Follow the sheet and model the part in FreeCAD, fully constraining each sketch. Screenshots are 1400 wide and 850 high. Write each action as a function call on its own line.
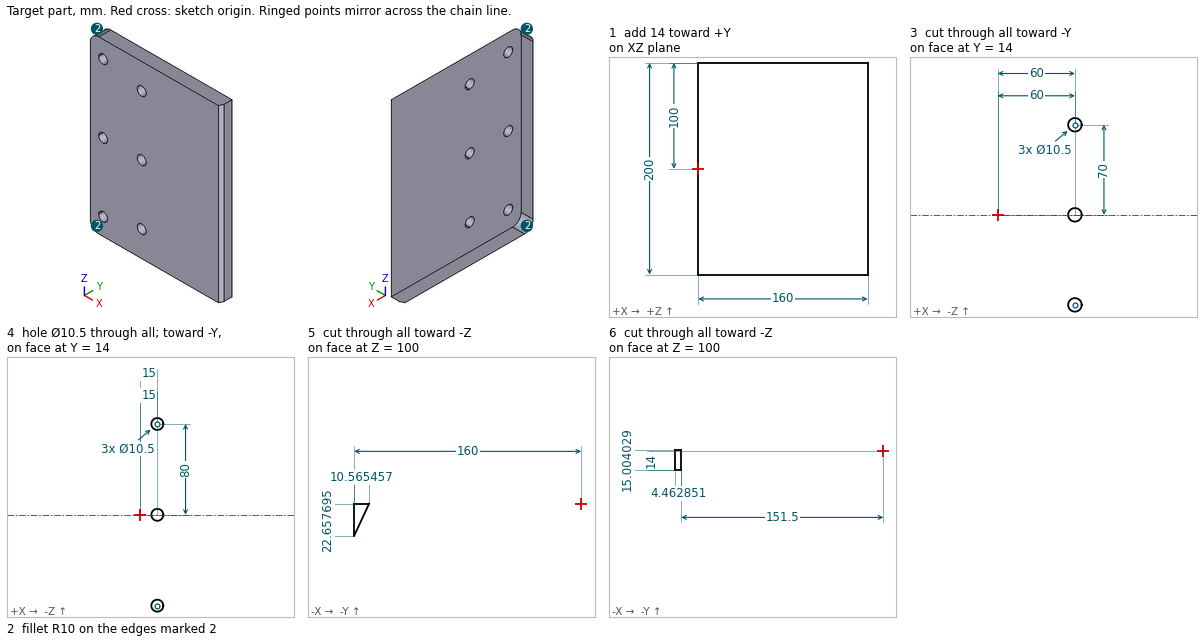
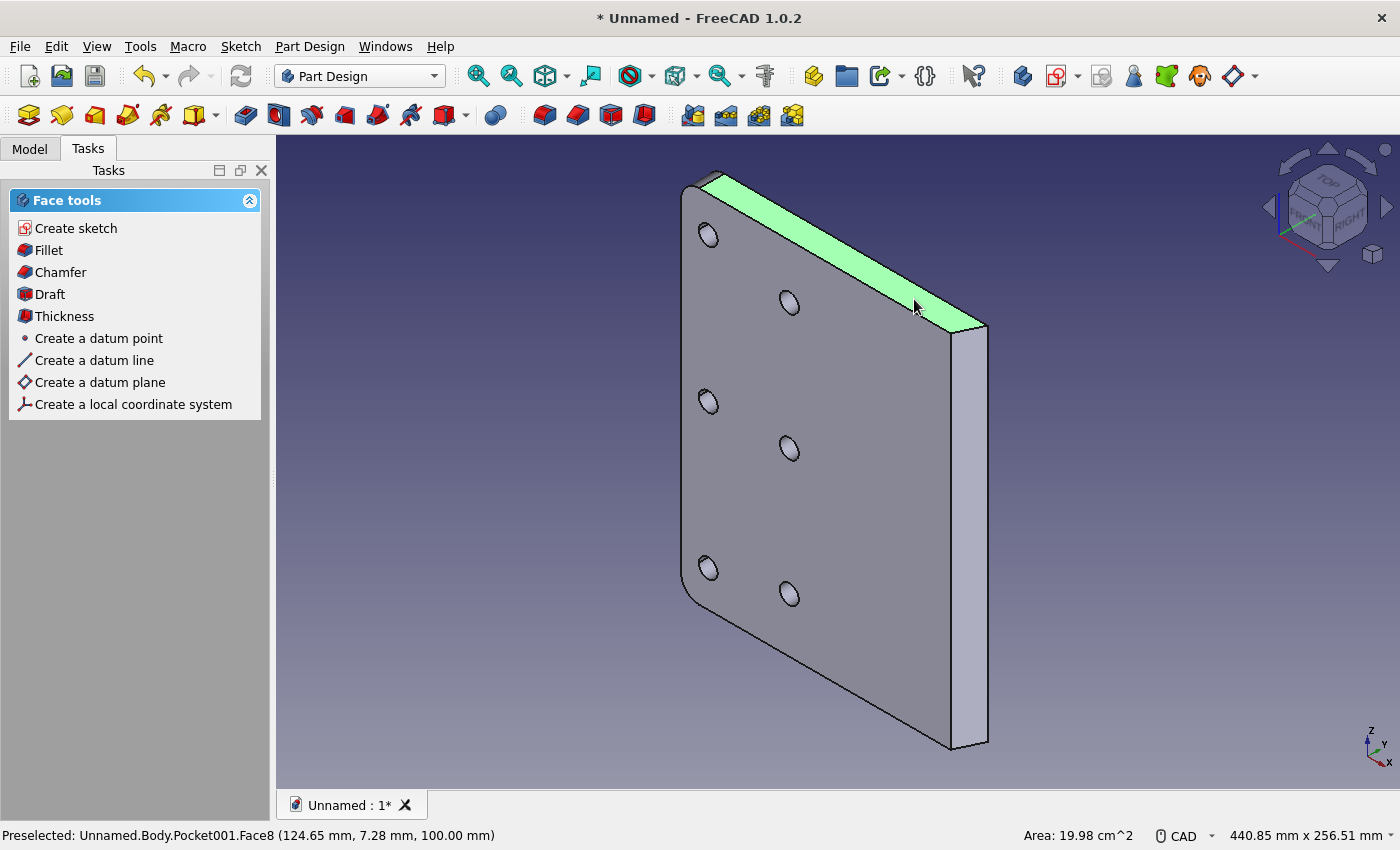
click(1056, 76)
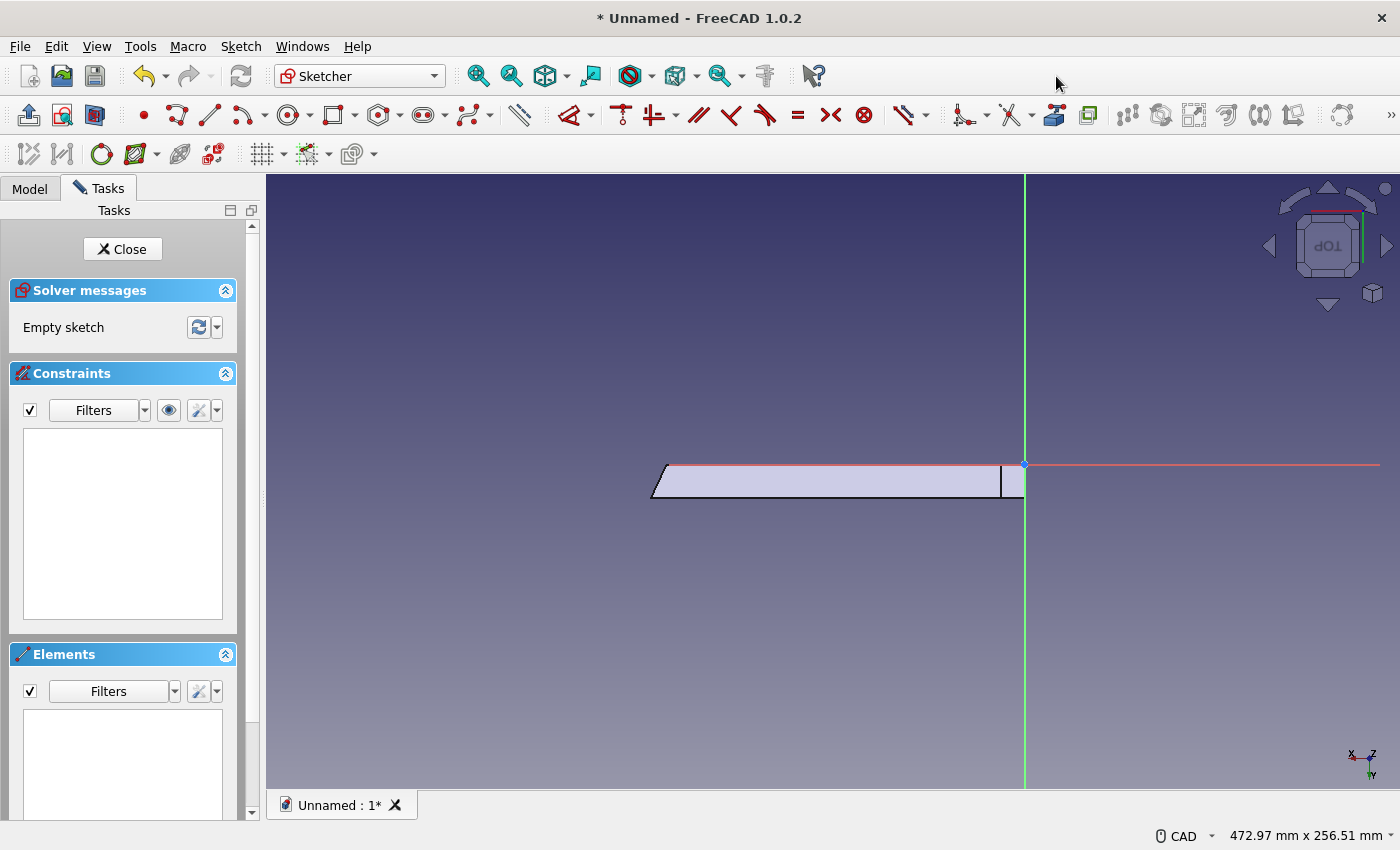
scroll(645, 480, up, 12)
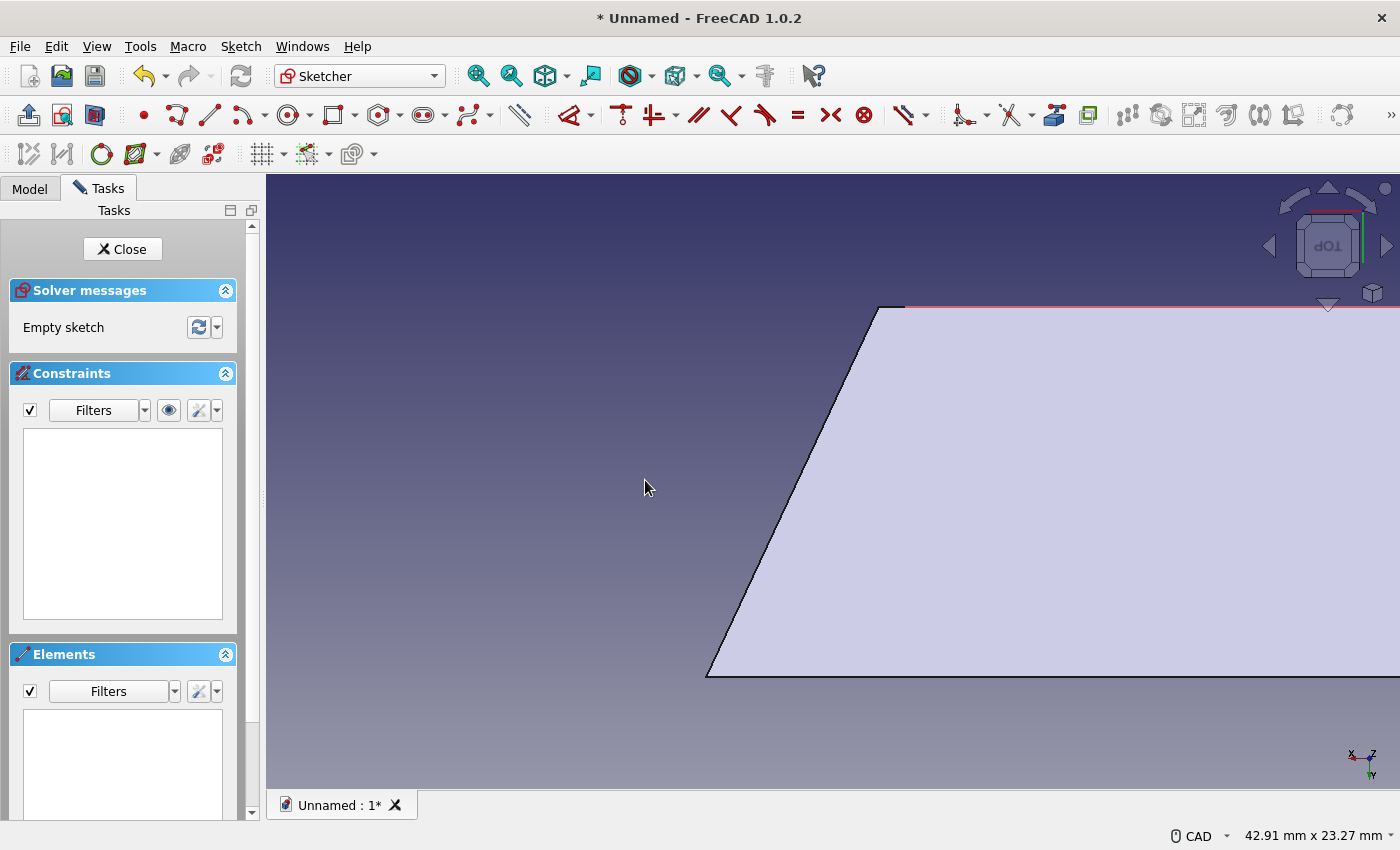
click(332, 116)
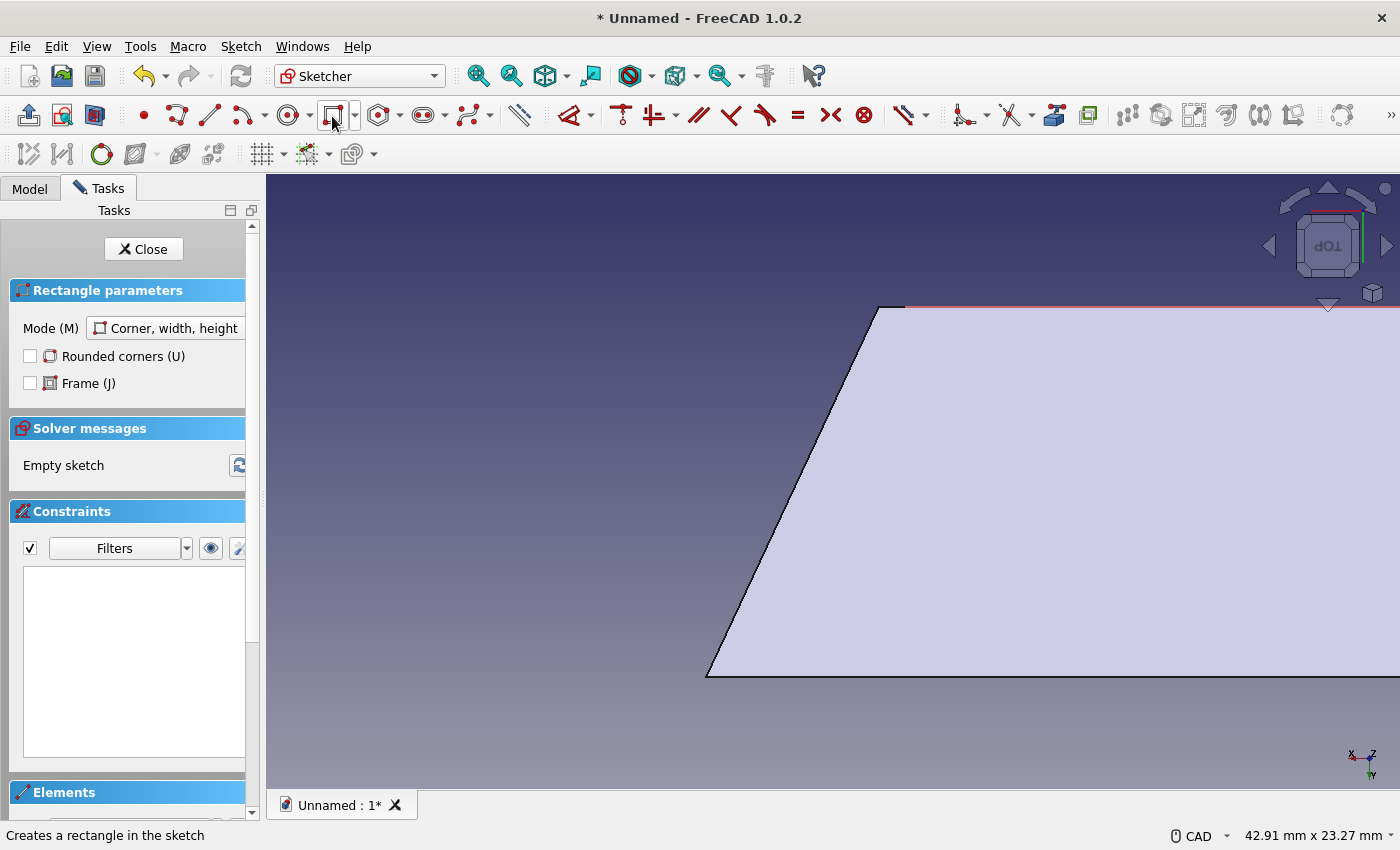
click(706, 280)
click(824, 677)
key(Escape)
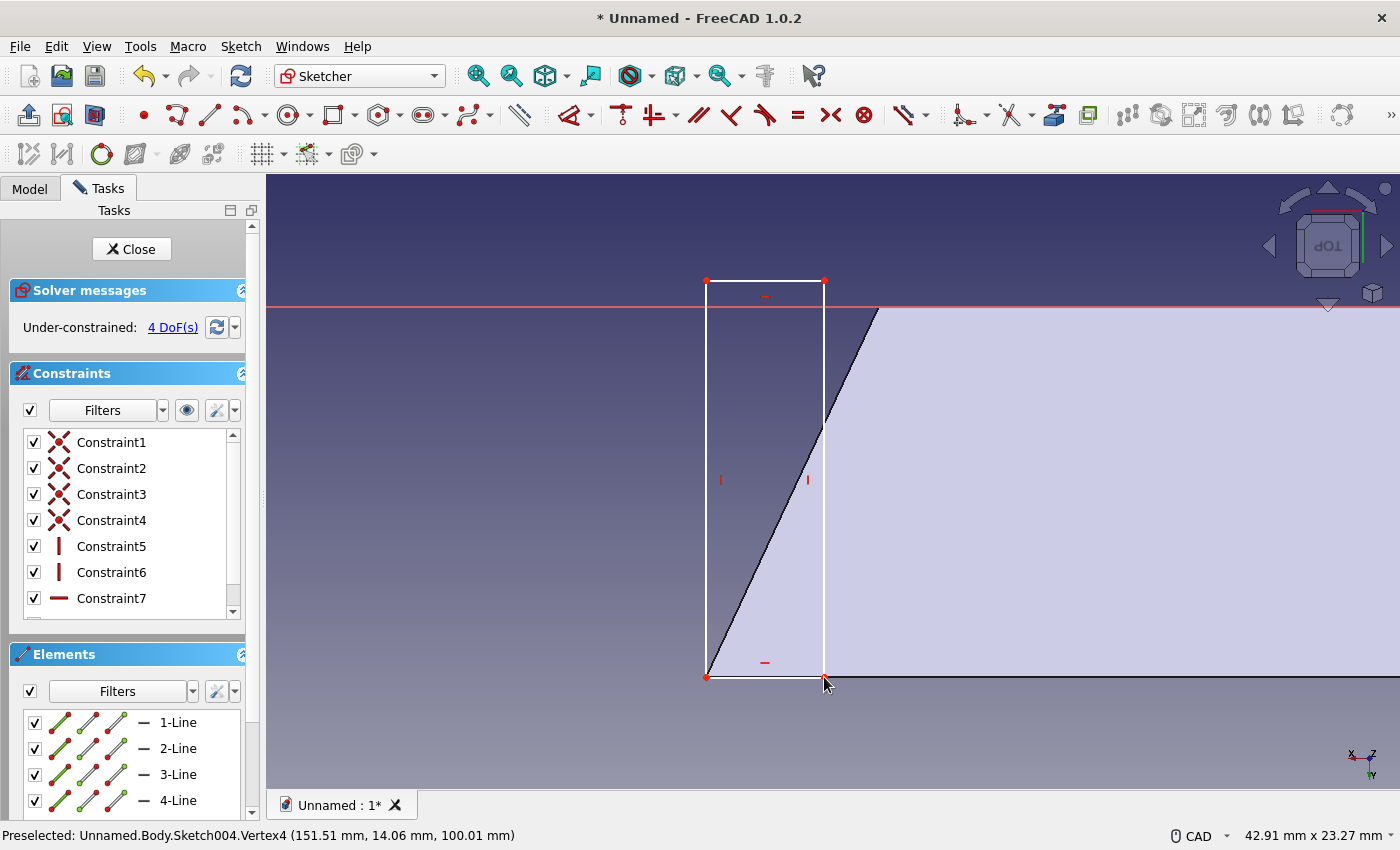
key(d)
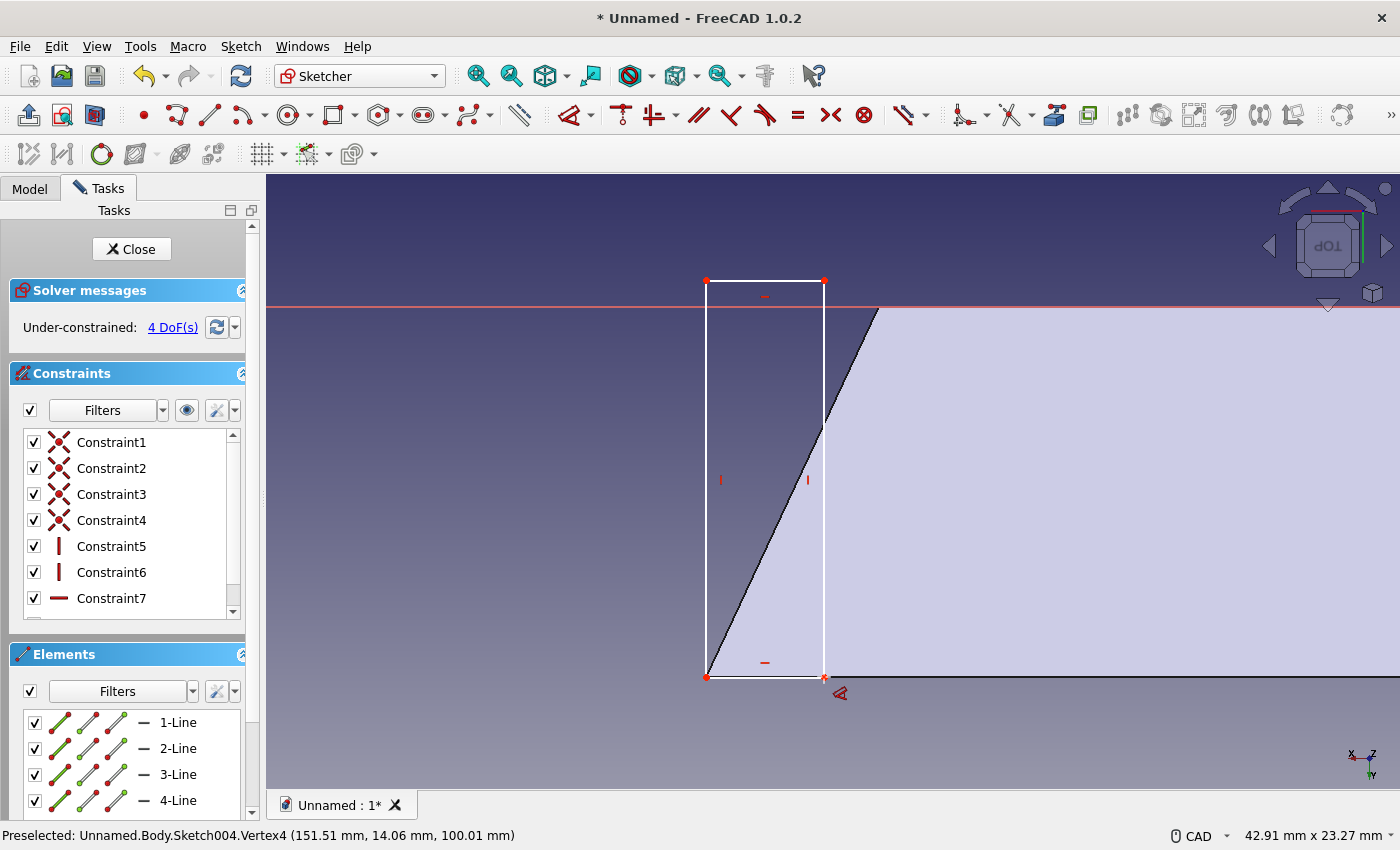
click(706, 678)
click(672, 492)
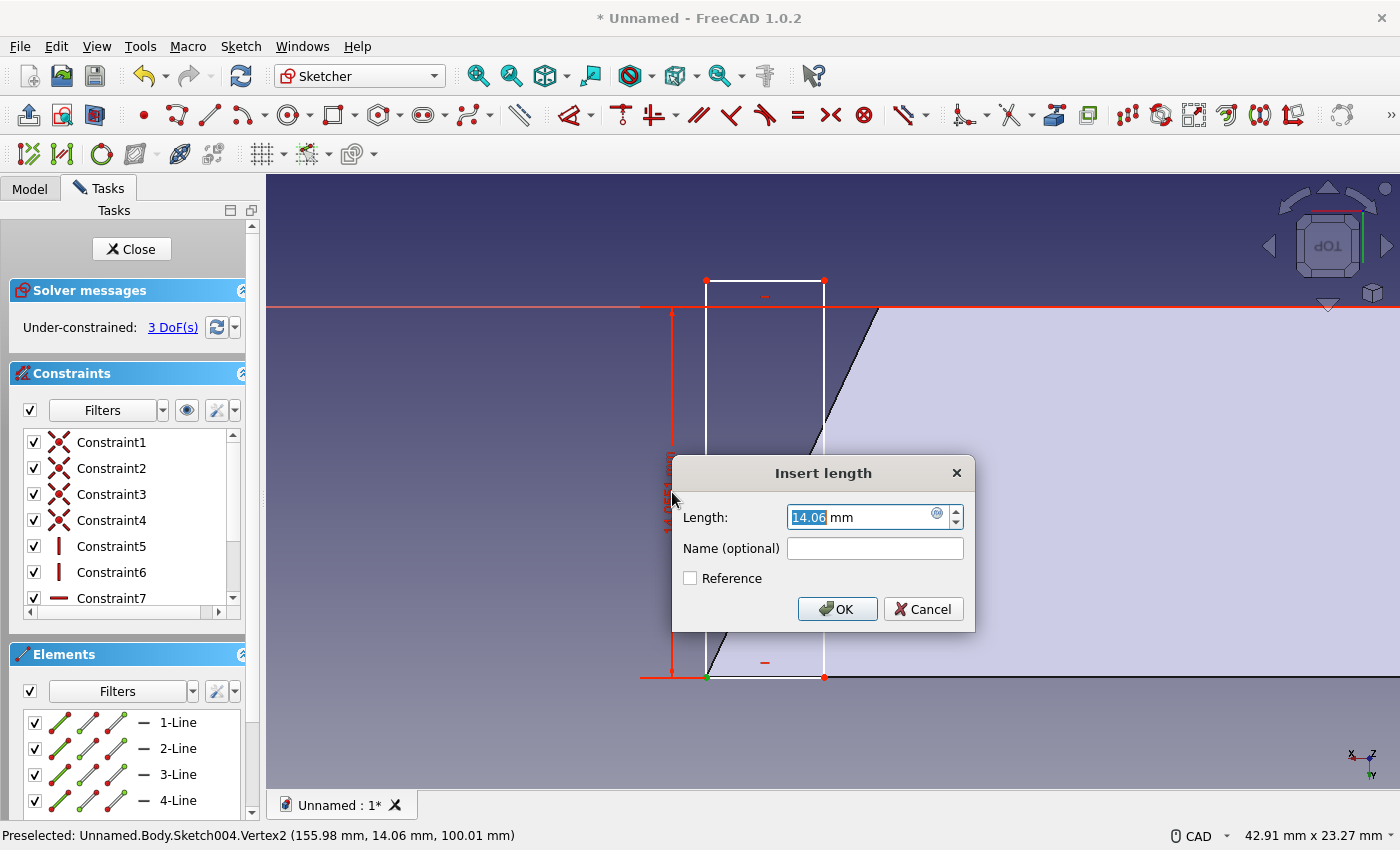
text(14)
key(Return)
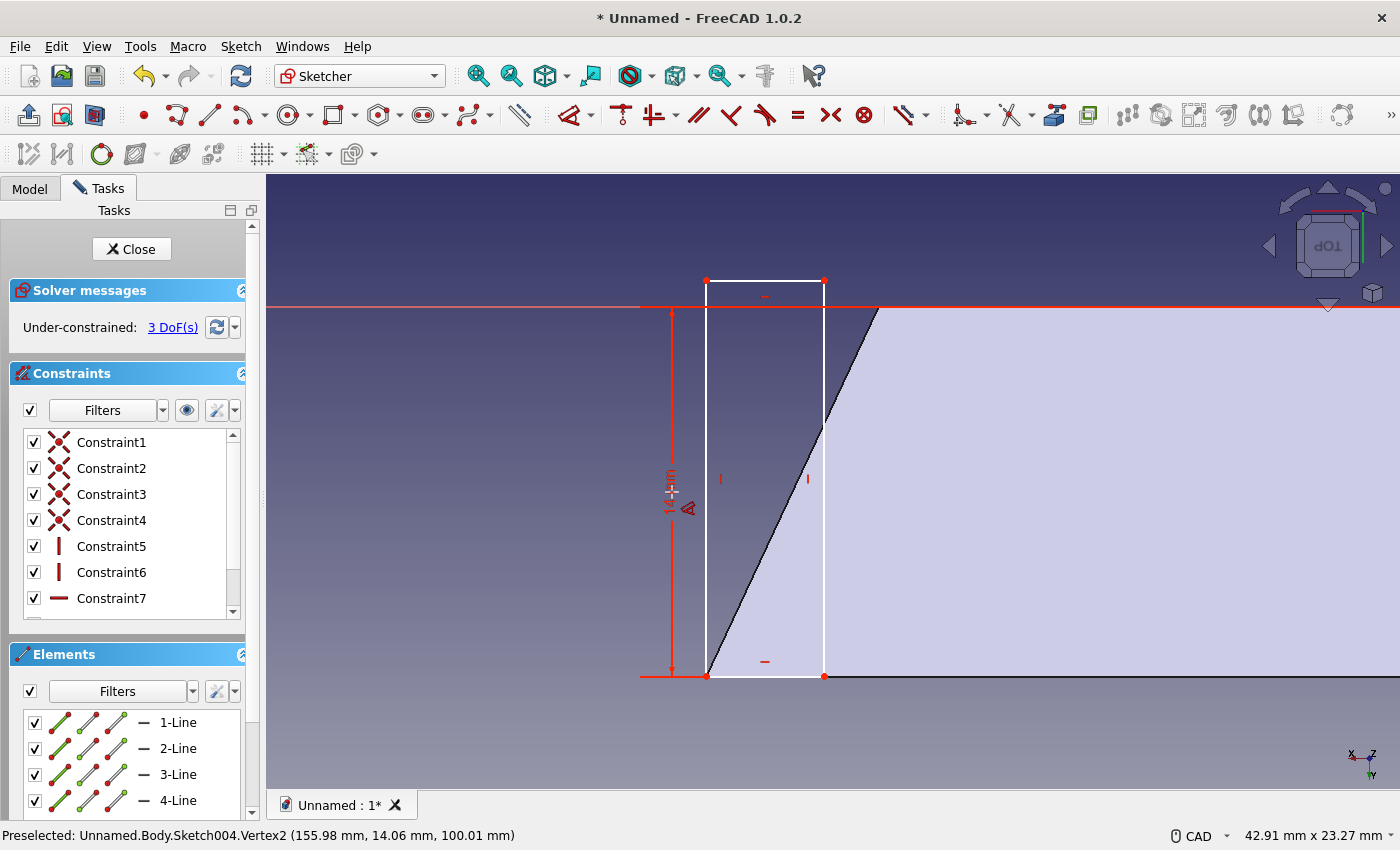
click(824, 677)
click(1030, 711)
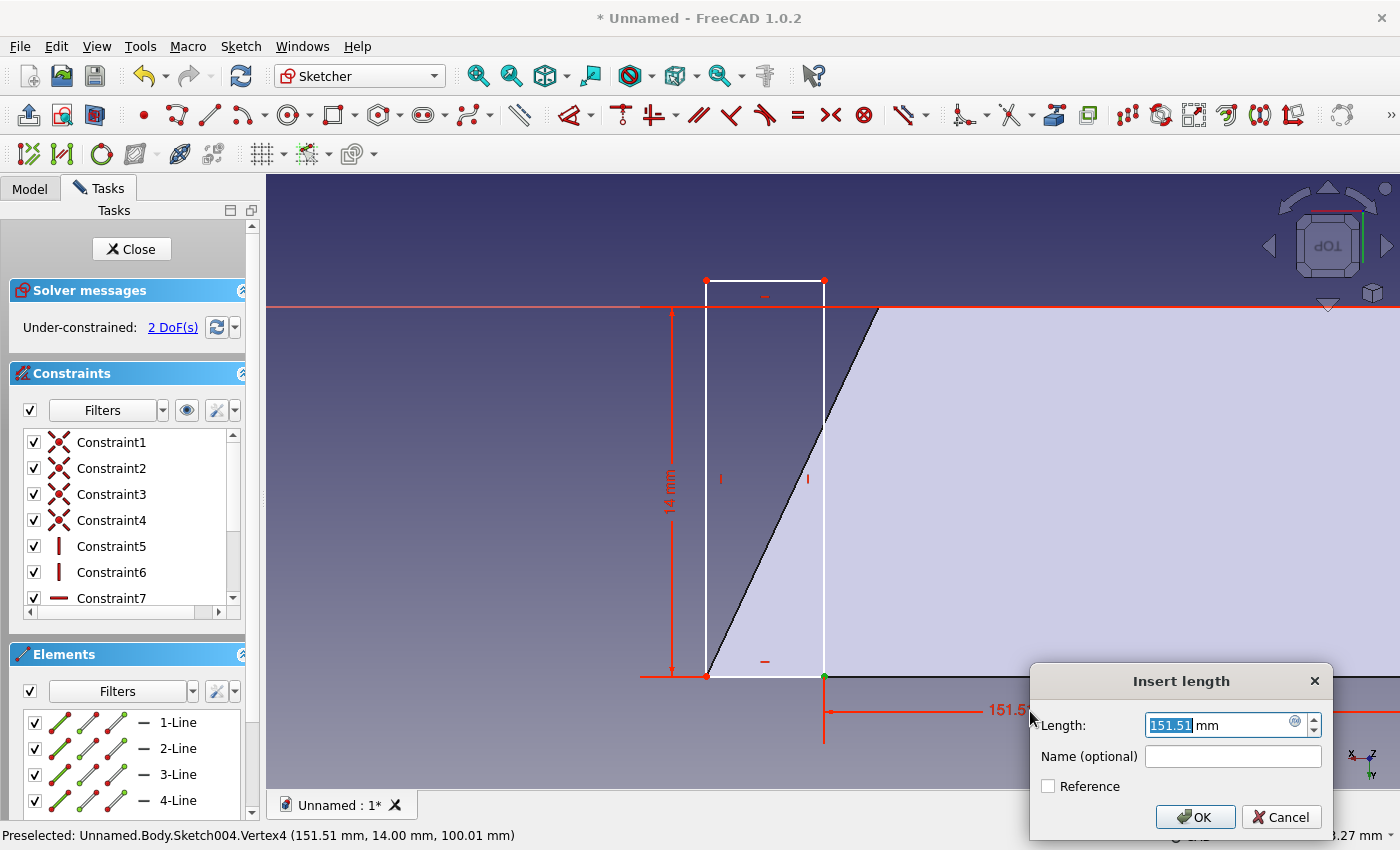
text(151.5)
key(Return)